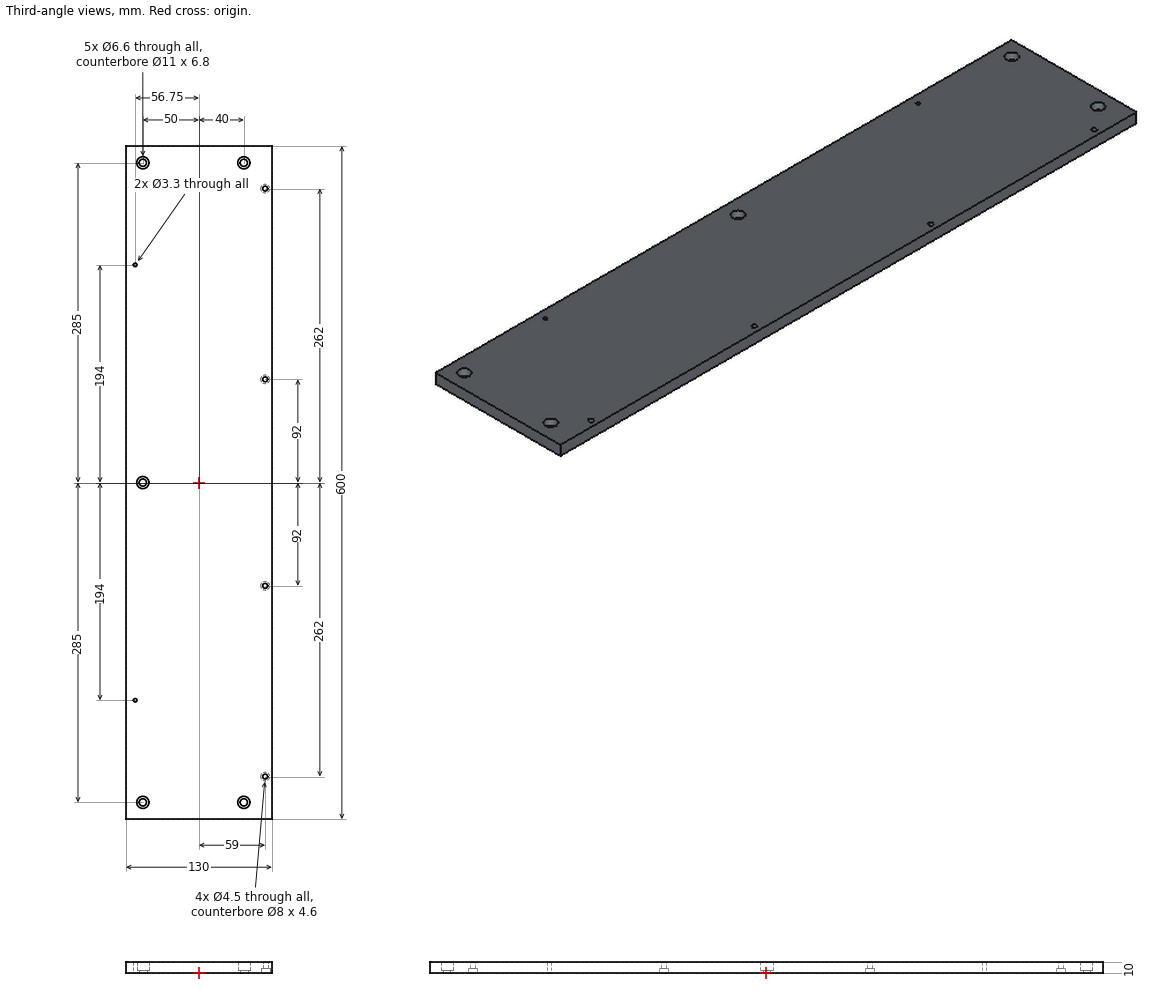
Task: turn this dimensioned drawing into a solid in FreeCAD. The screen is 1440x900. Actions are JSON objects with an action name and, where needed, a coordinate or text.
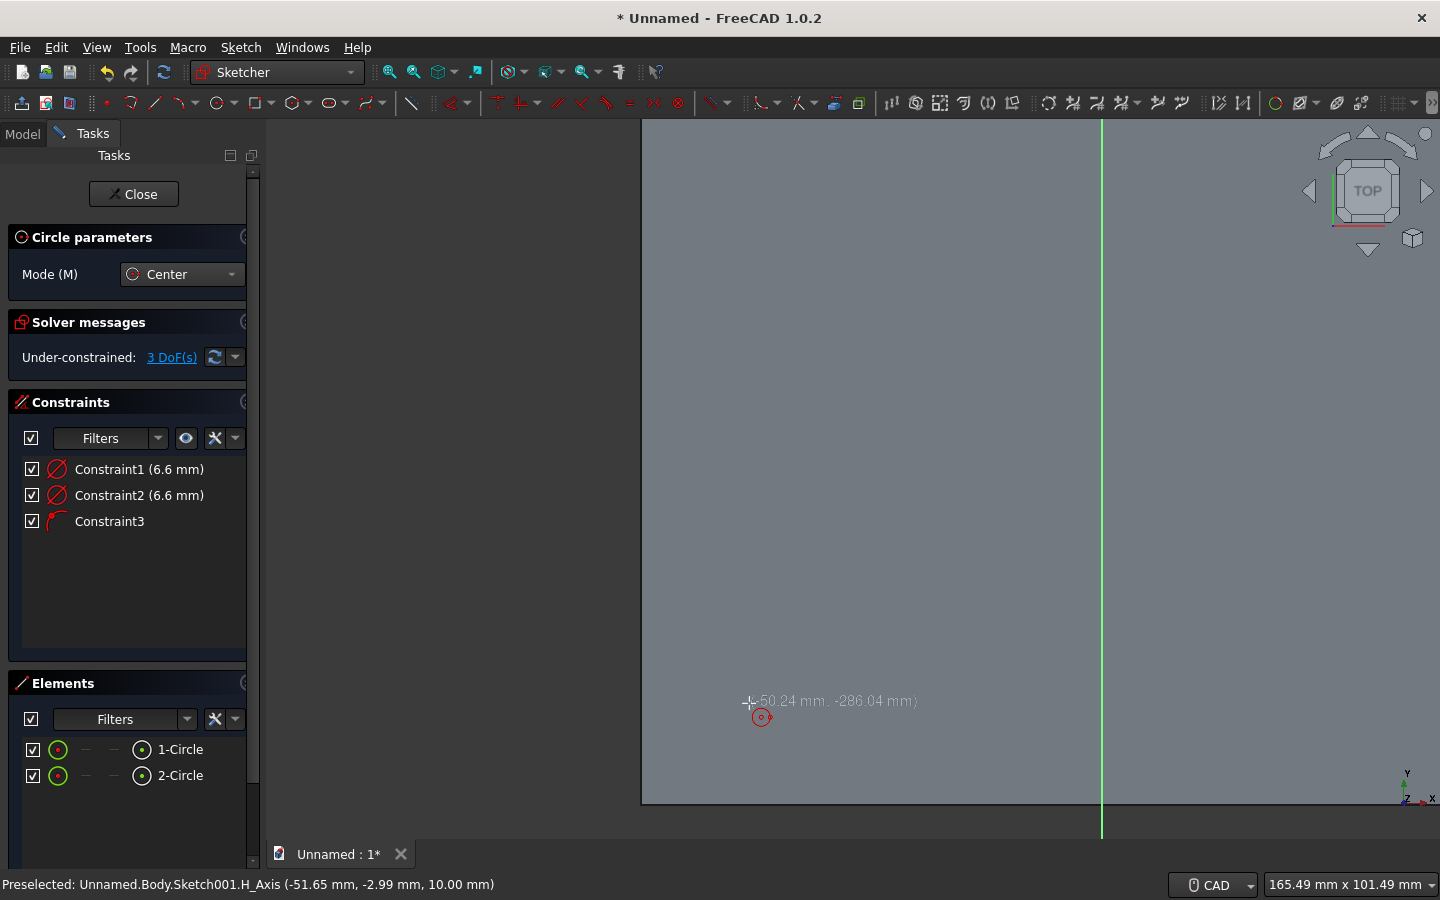
{"action": "scroll", "coordinate": [749, 704], "scroll_direction": "down", "scroll_amount": 11}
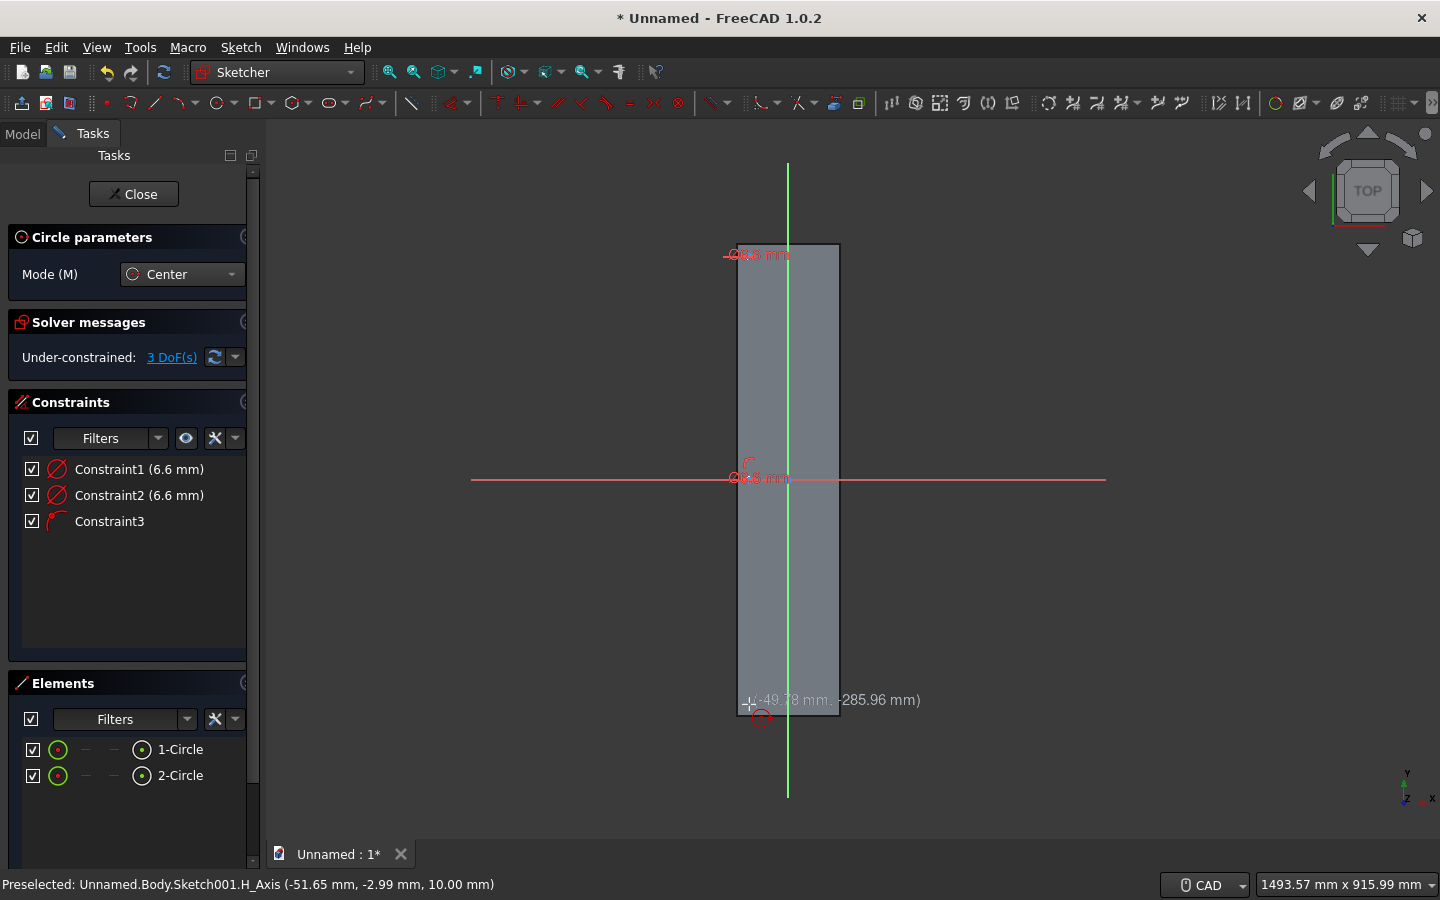
{"action": "left_click", "coordinate": [749, 704]}
{"action": "mouse_move", "coordinate": [751, 702]}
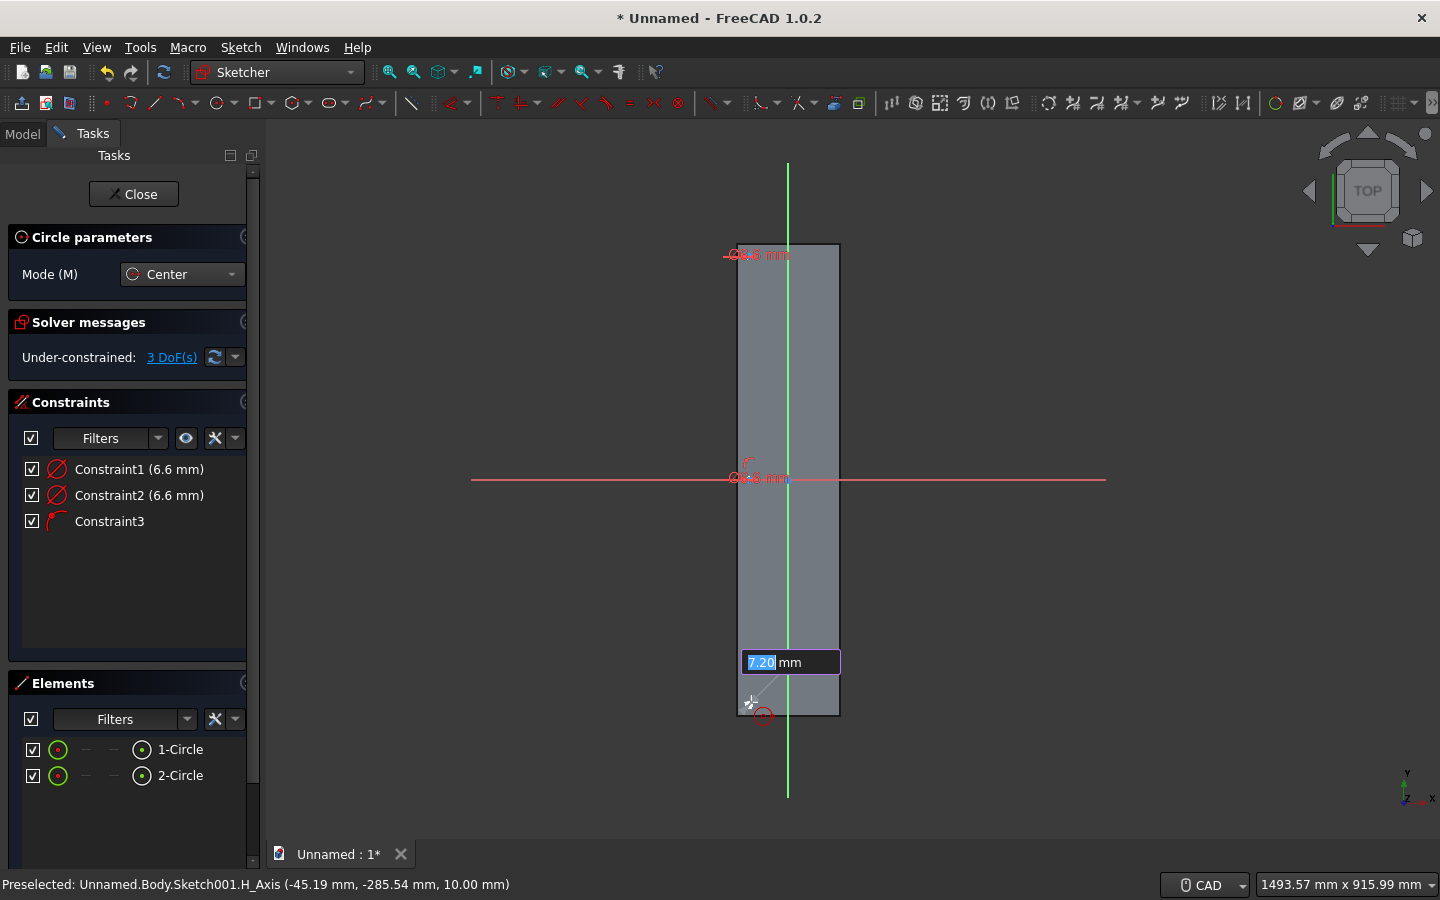
{"action": "type", "text": "6.6"}
{"action": "key", "text": "Return"}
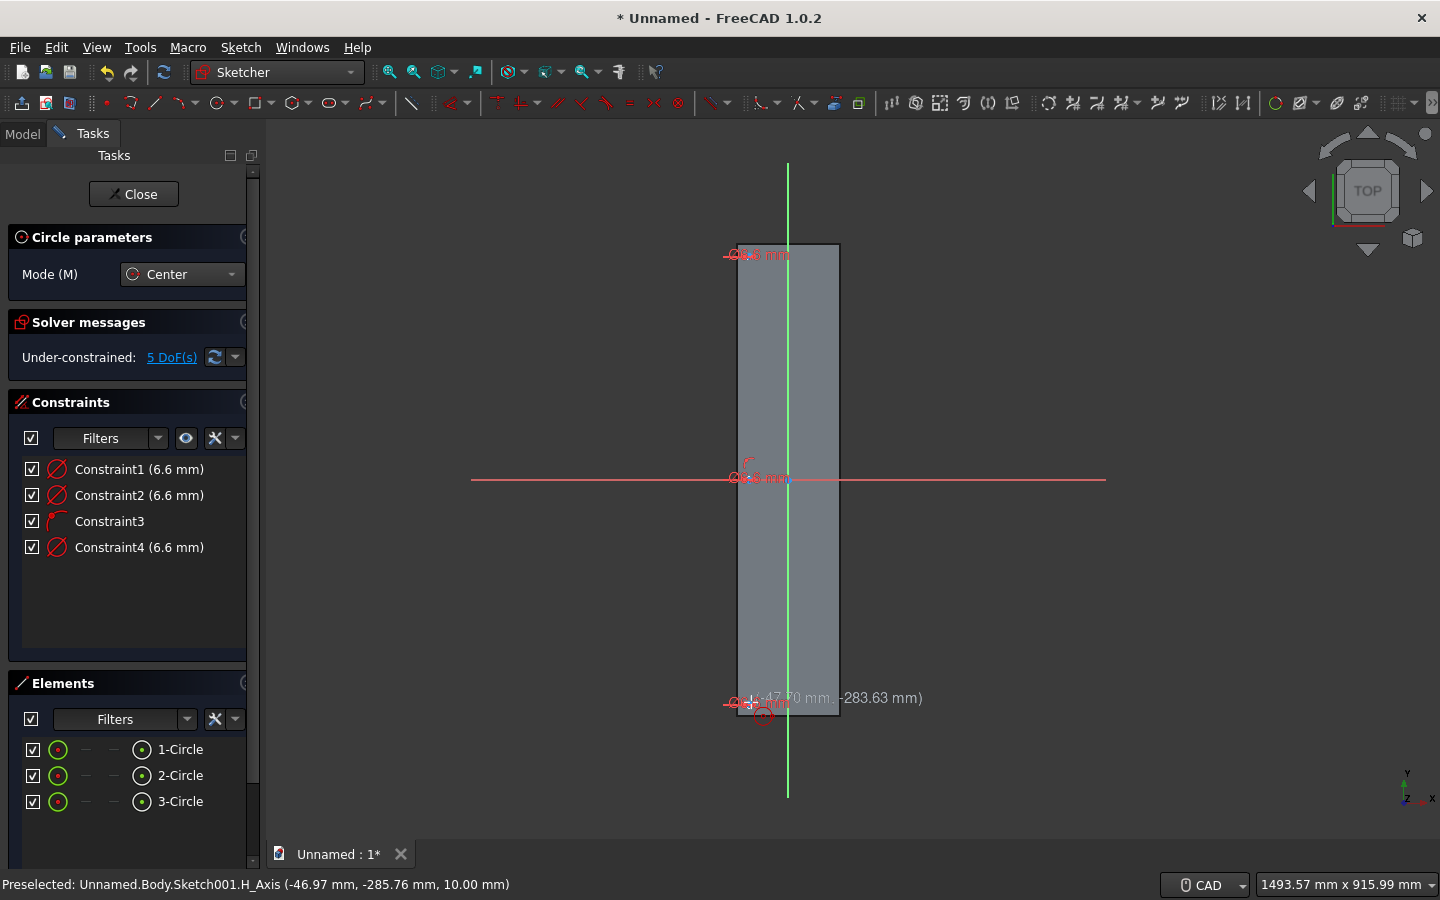
{"action": "scroll", "coordinate": [820, 256], "scroll_direction": "up", "scroll_amount": 11}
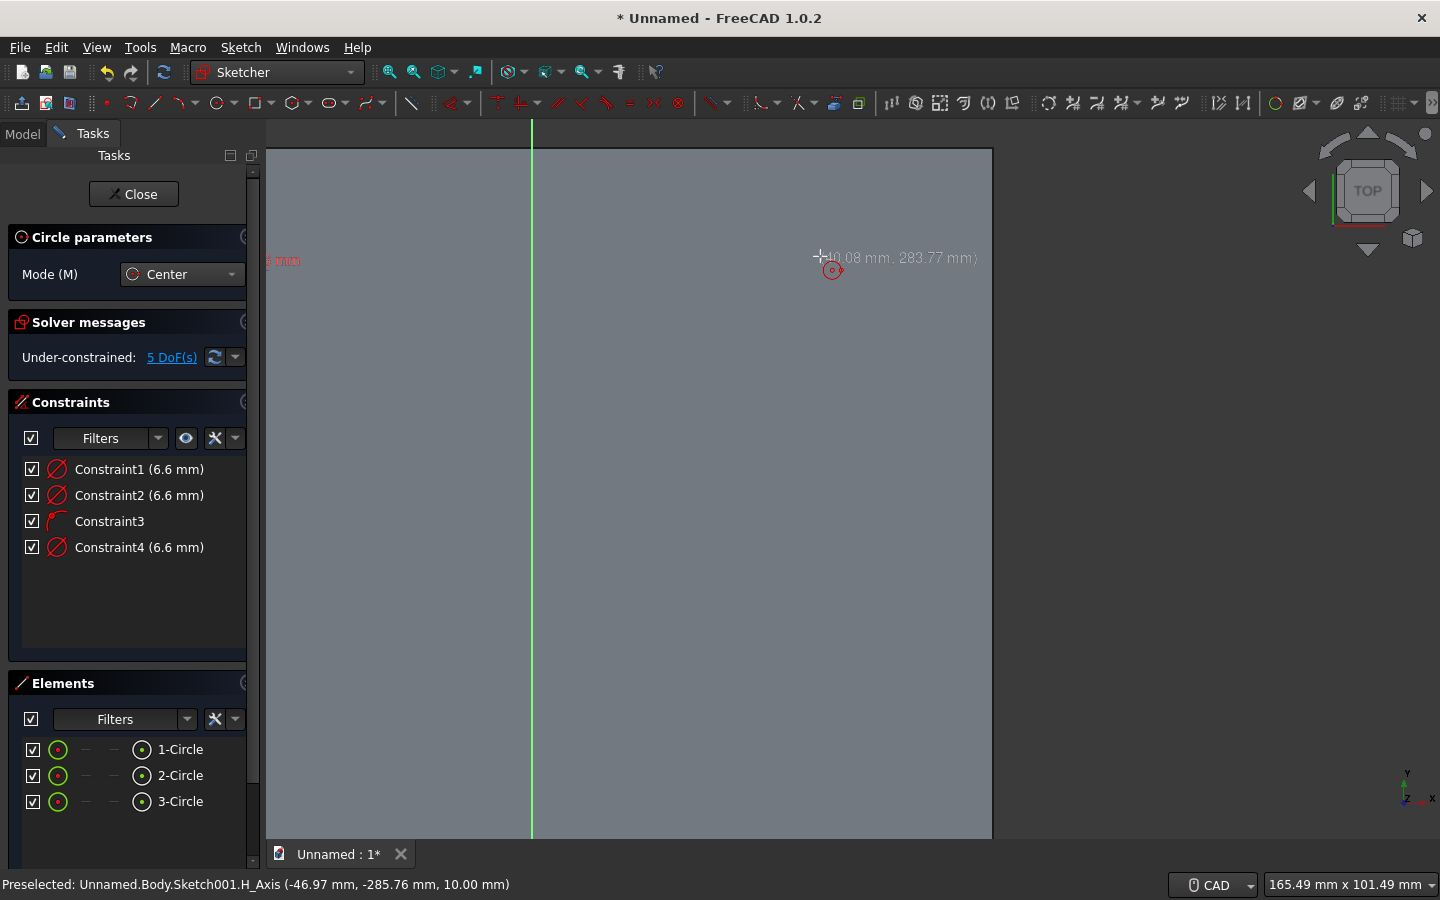
{"action": "scroll", "coordinate": [820, 255], "scroll_direction": "down", "scroll_amount": 11}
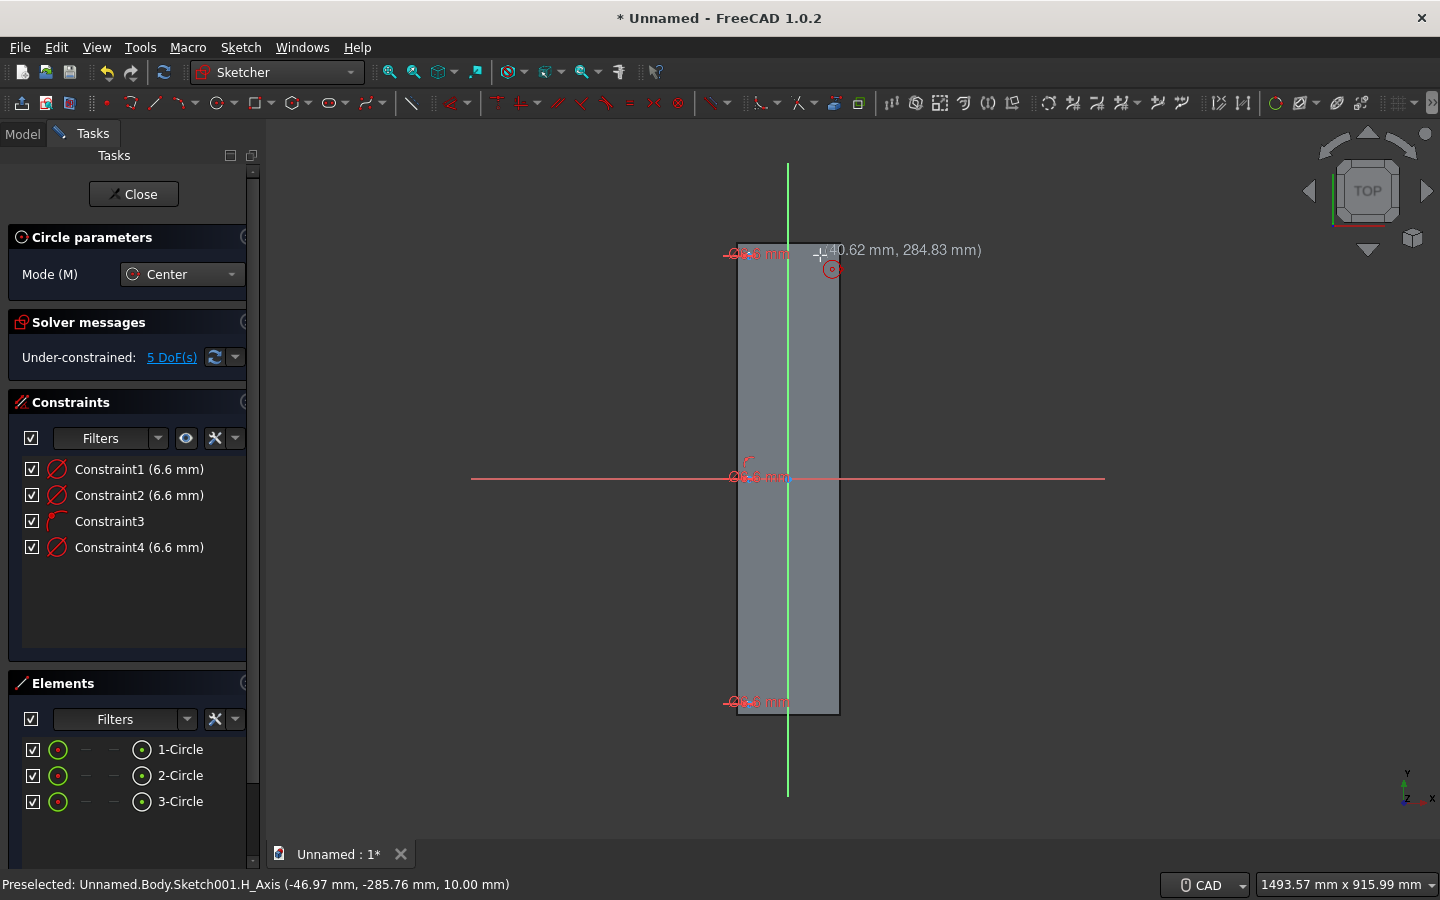
{"action": "left_click", "coordinate": [820, 255]}
{"action": "mouse_move", "coordinate": [822, 253]}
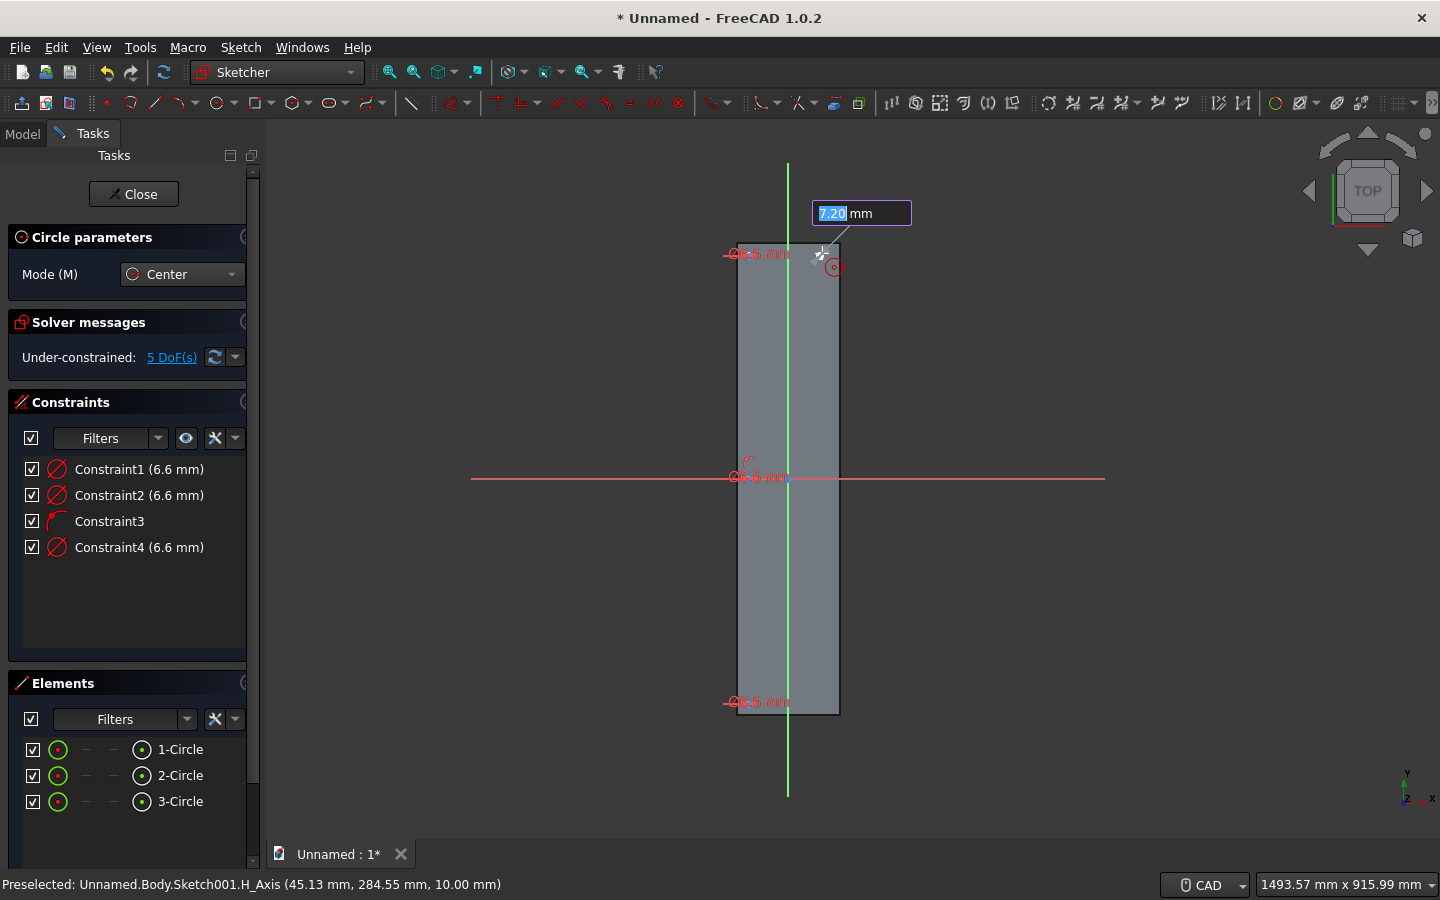
{"action": "type", "text": "6.6"}
{"action": "key", "text": "Return"}